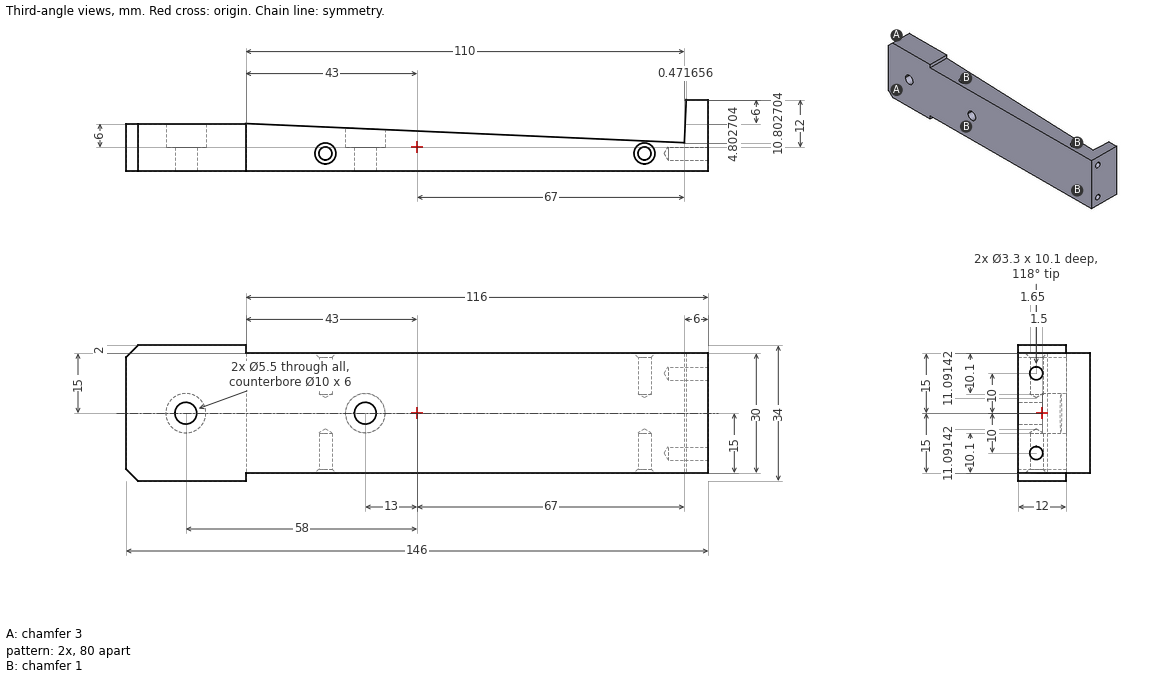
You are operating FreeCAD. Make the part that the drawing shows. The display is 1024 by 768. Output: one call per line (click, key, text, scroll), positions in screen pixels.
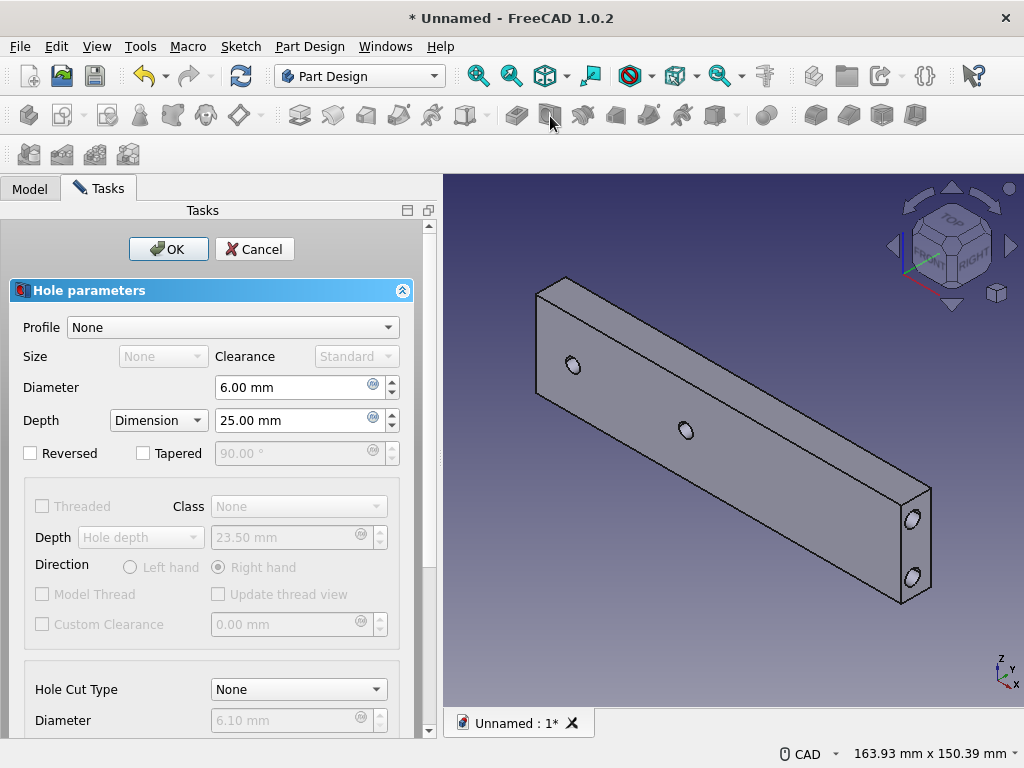
triple_click(300, 388)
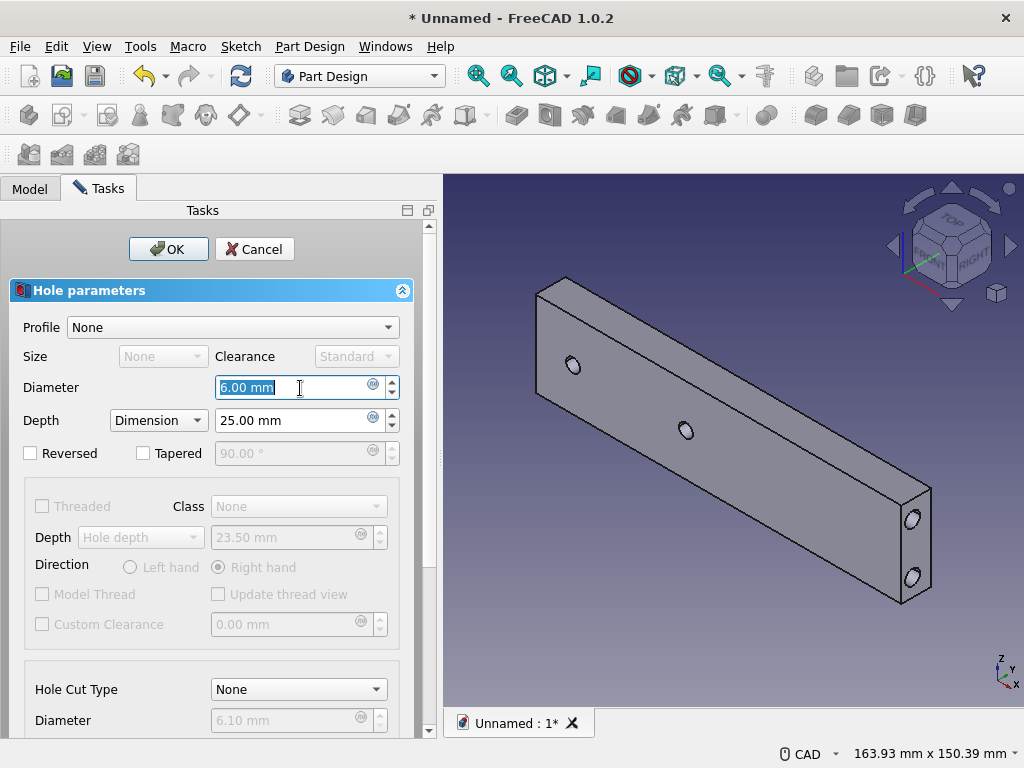
text(3.3)
key(Tab)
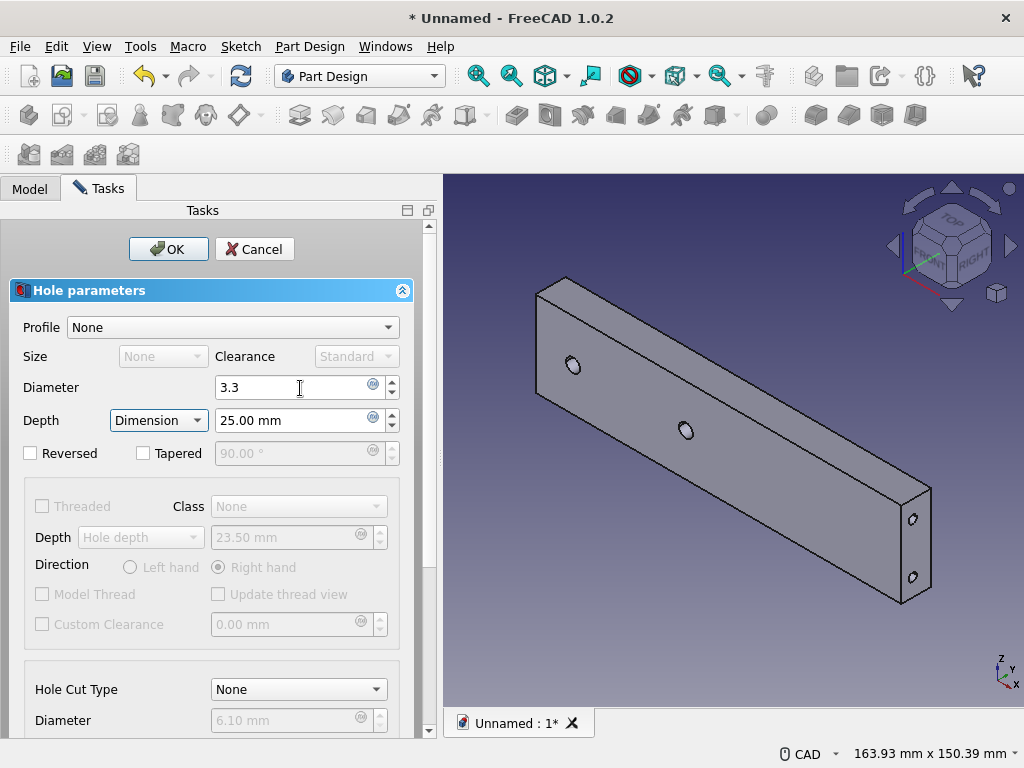
triple_click(300, 420)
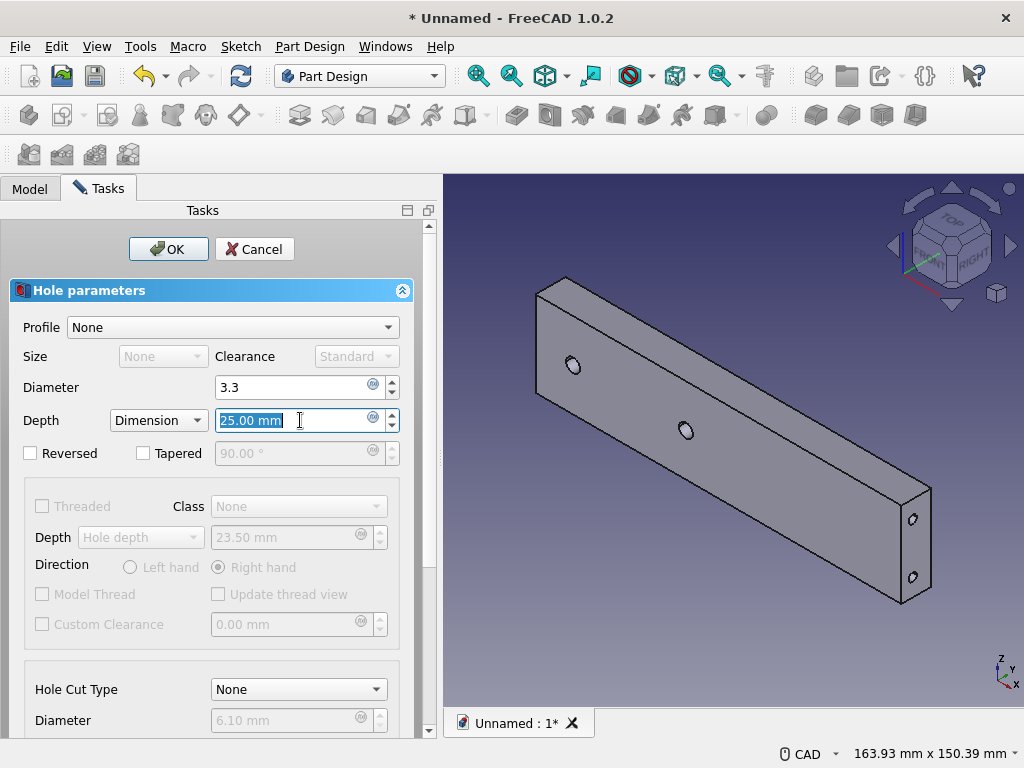
text(10.1)
key(Tab)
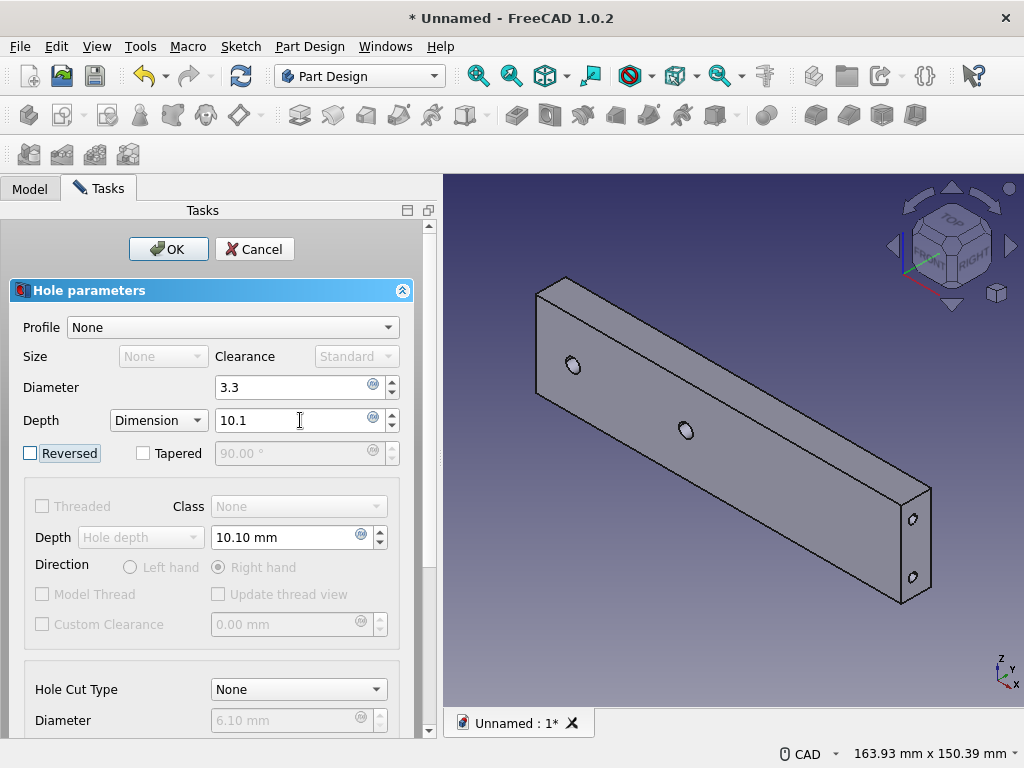
click(169, 249)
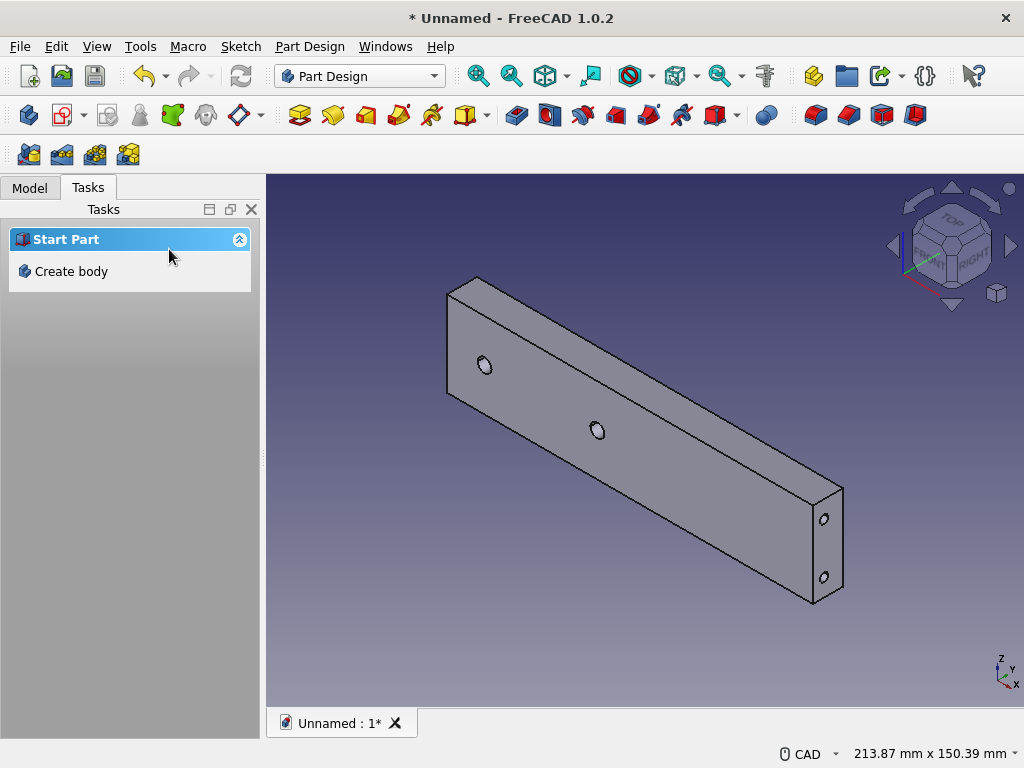
key(2)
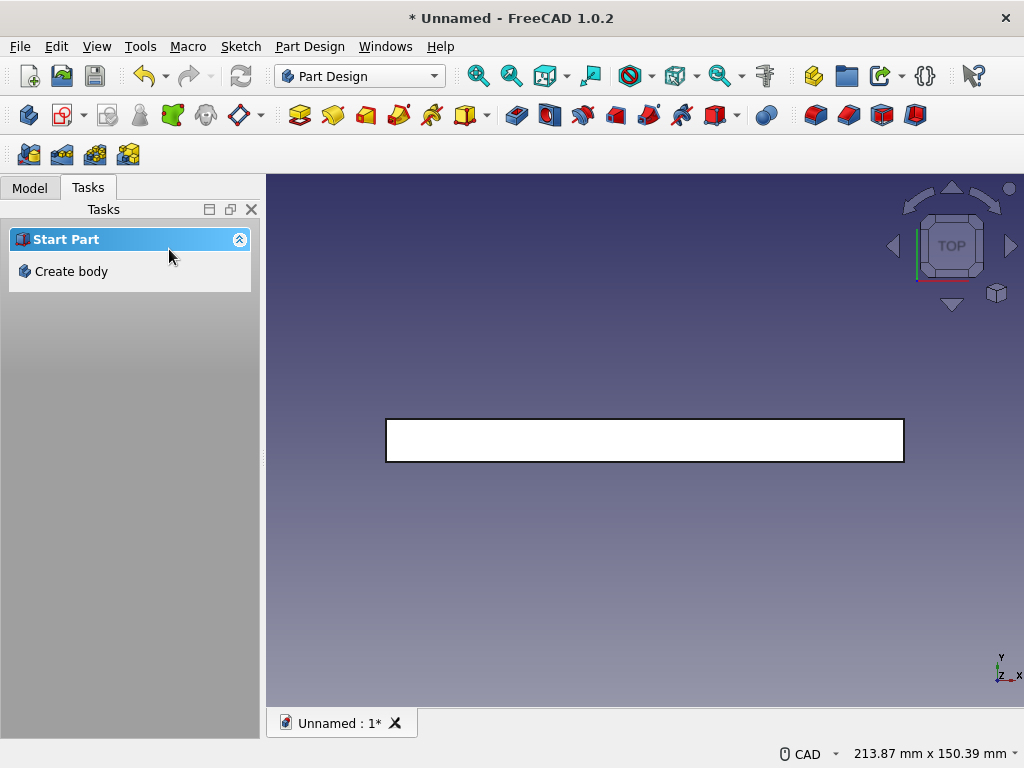
click(386, 439)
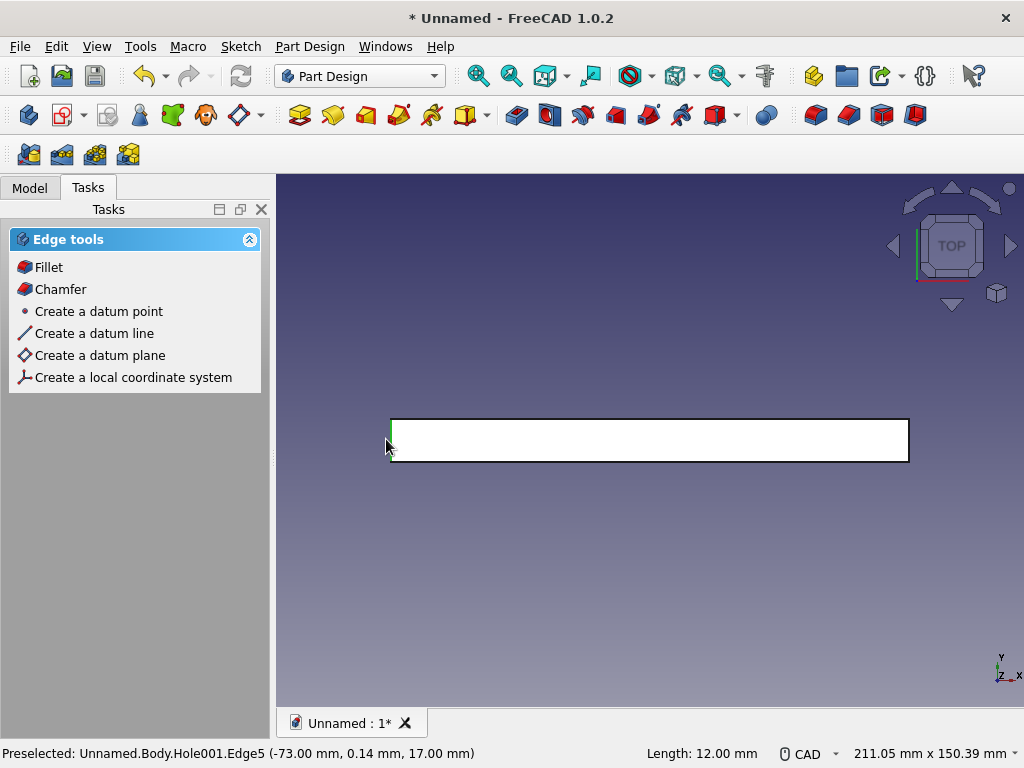
key(0)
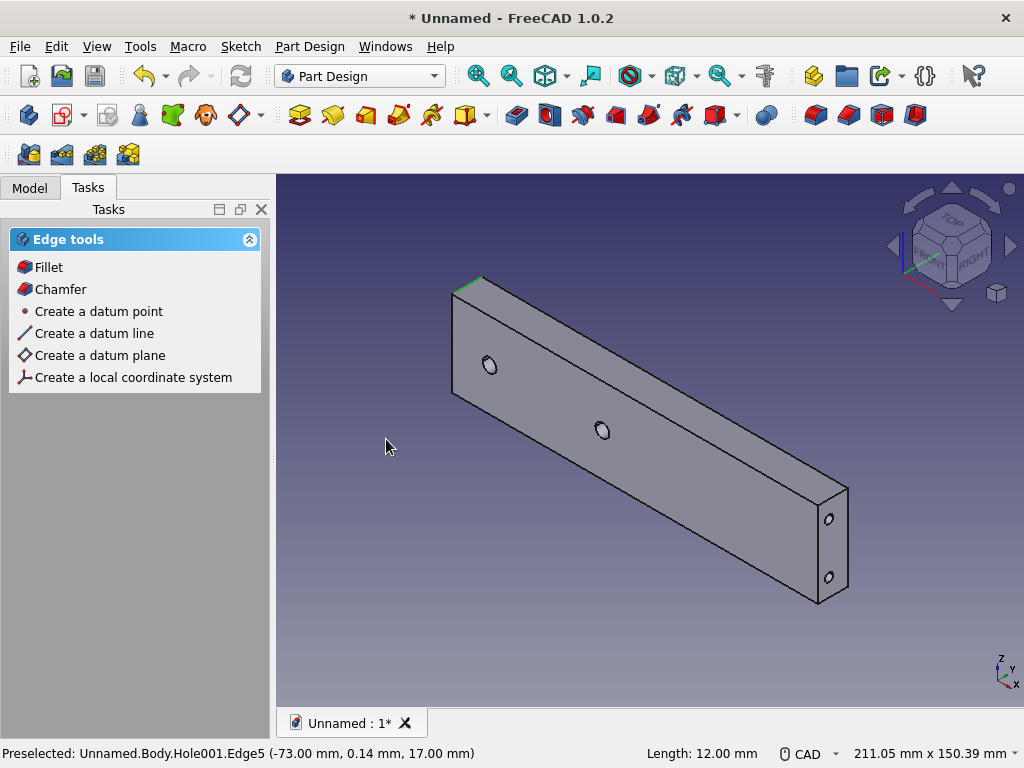
key(1)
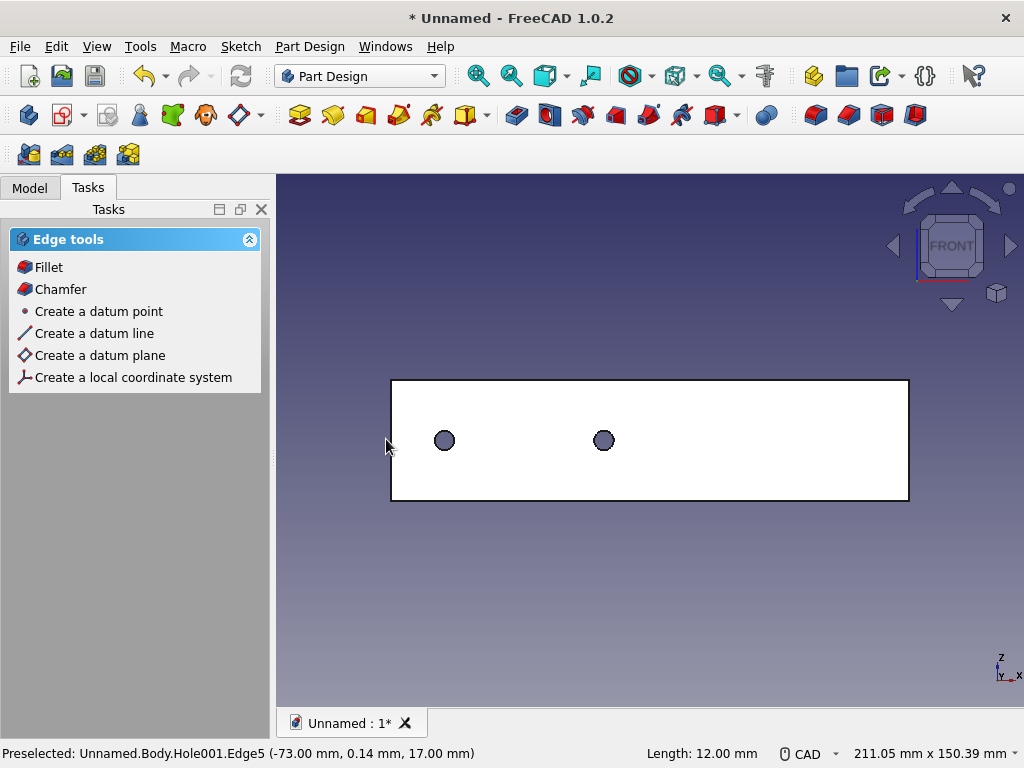
key(3)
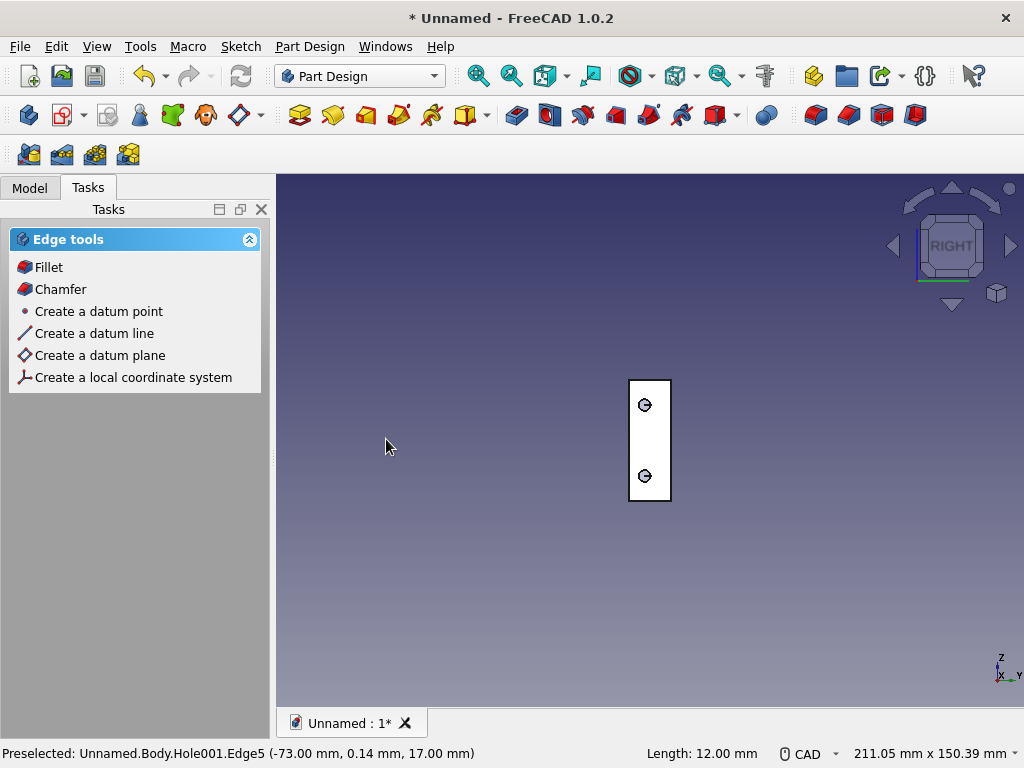
click(479, 76)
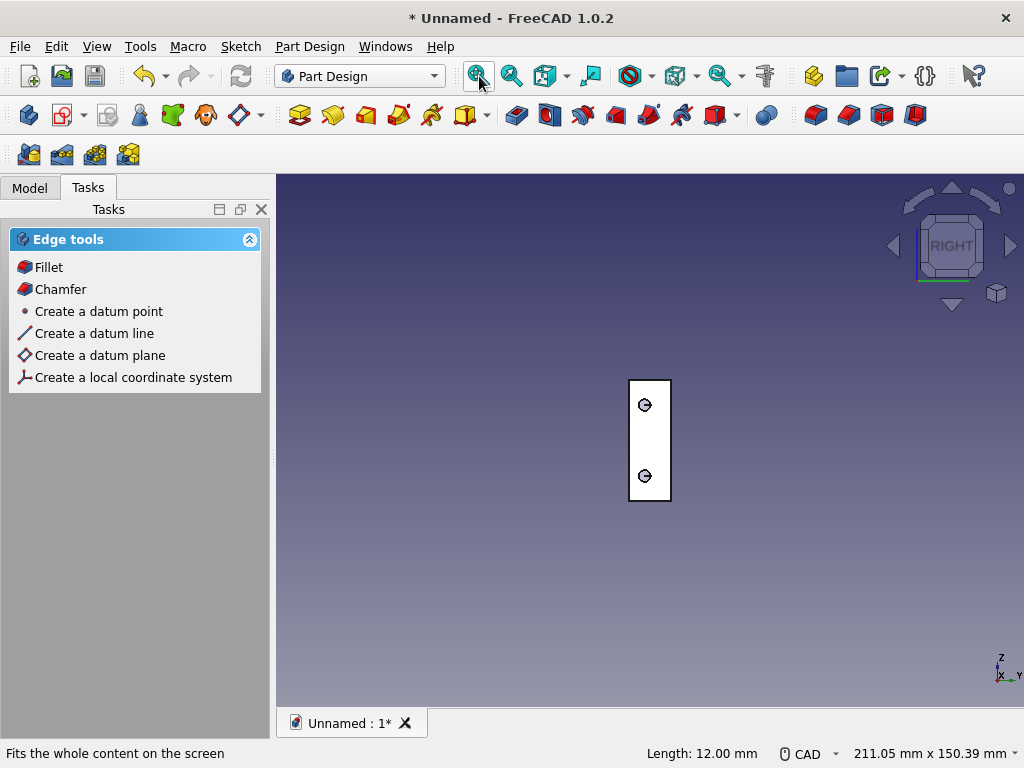
key(5)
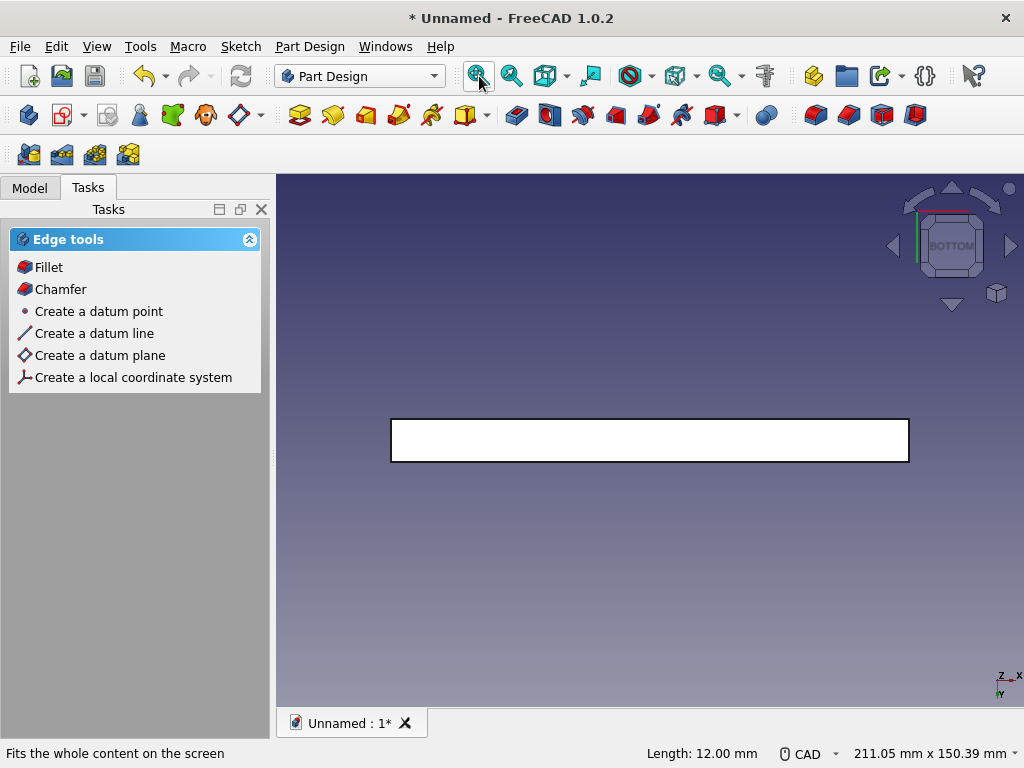
click(391, 439, ctrl)